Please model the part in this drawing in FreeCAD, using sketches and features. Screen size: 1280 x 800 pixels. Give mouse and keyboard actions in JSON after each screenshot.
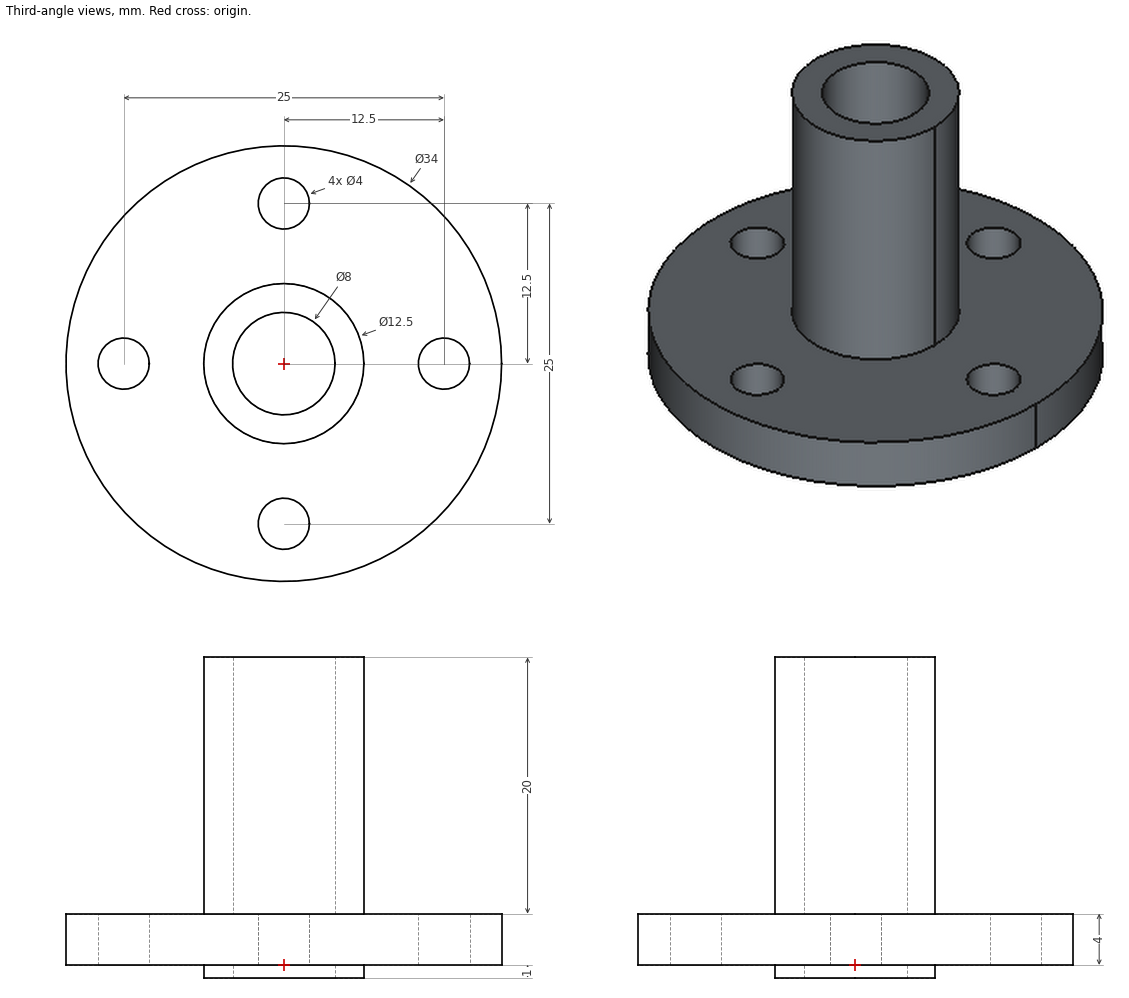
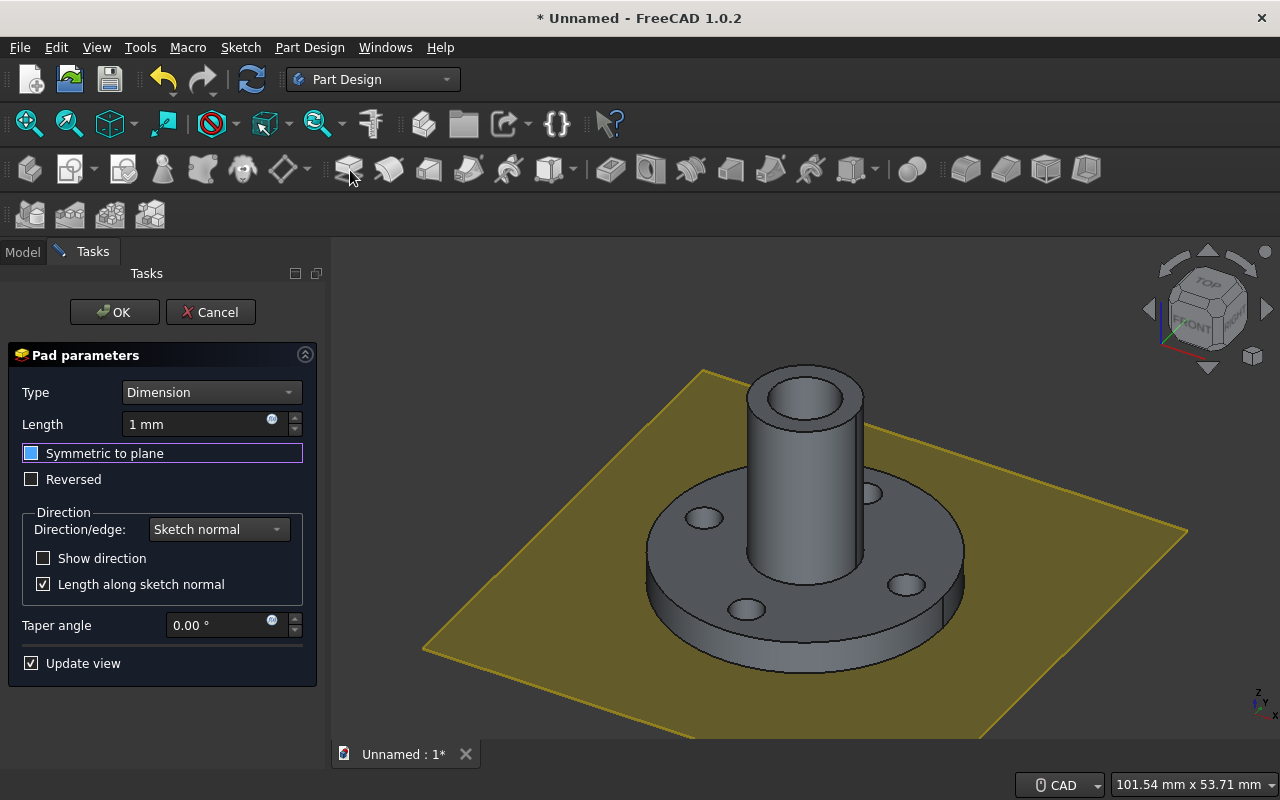
{"action": "left_click", "coordinate": [115, 312]}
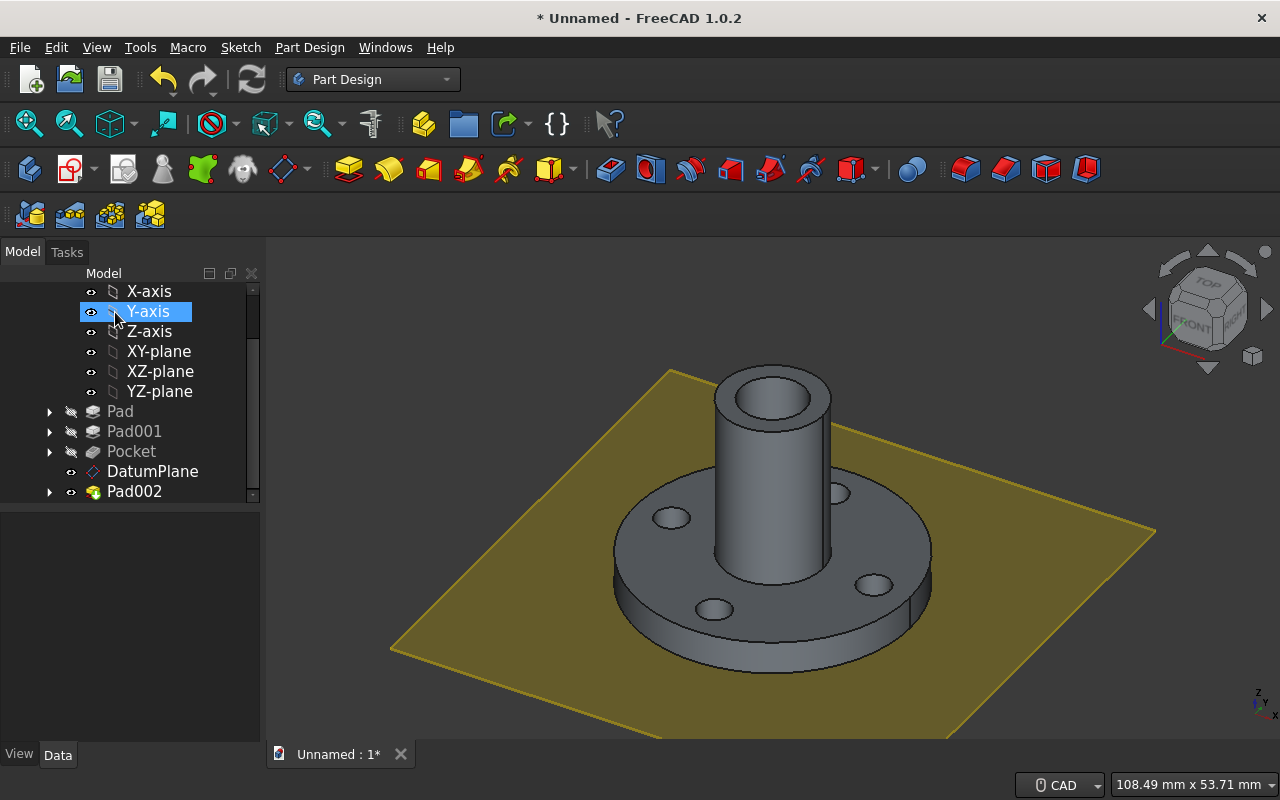
{"action": "left_click", "coordinate": [116, 472]}
{"action": "key", "text": "space"}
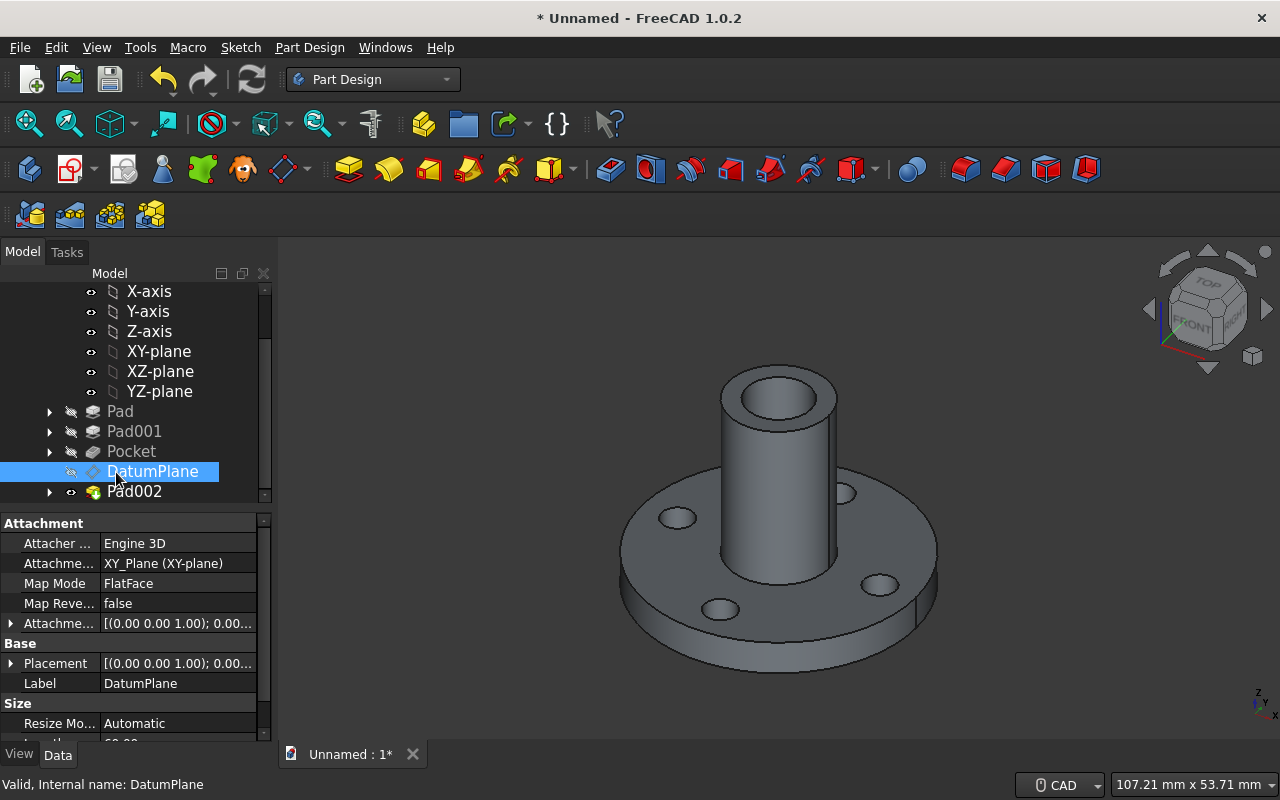
{"action": "key", "text": "0"}